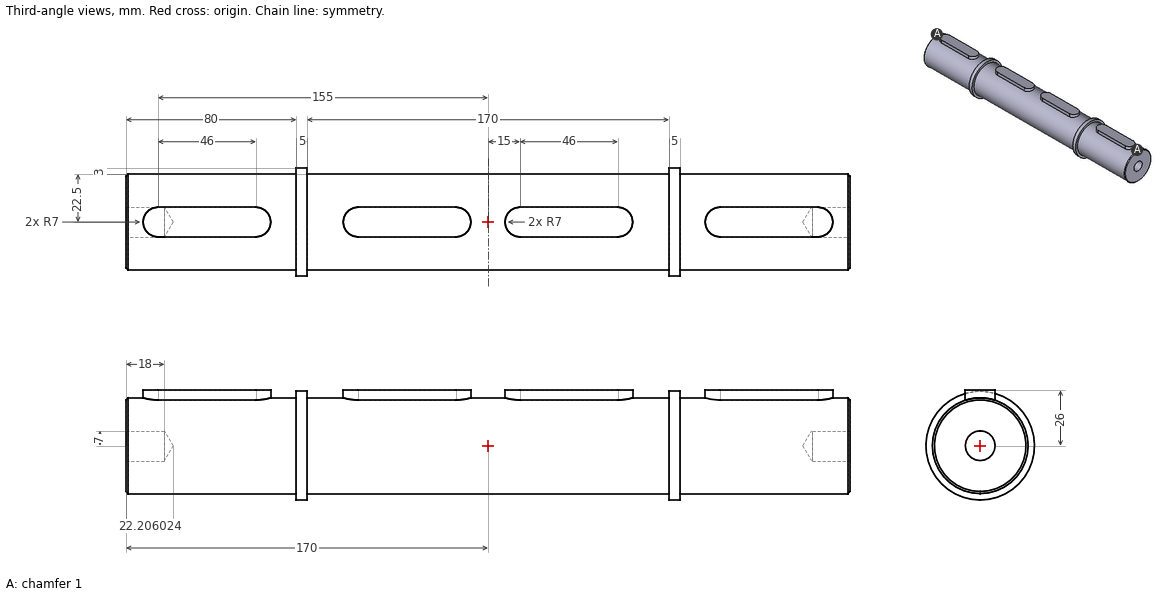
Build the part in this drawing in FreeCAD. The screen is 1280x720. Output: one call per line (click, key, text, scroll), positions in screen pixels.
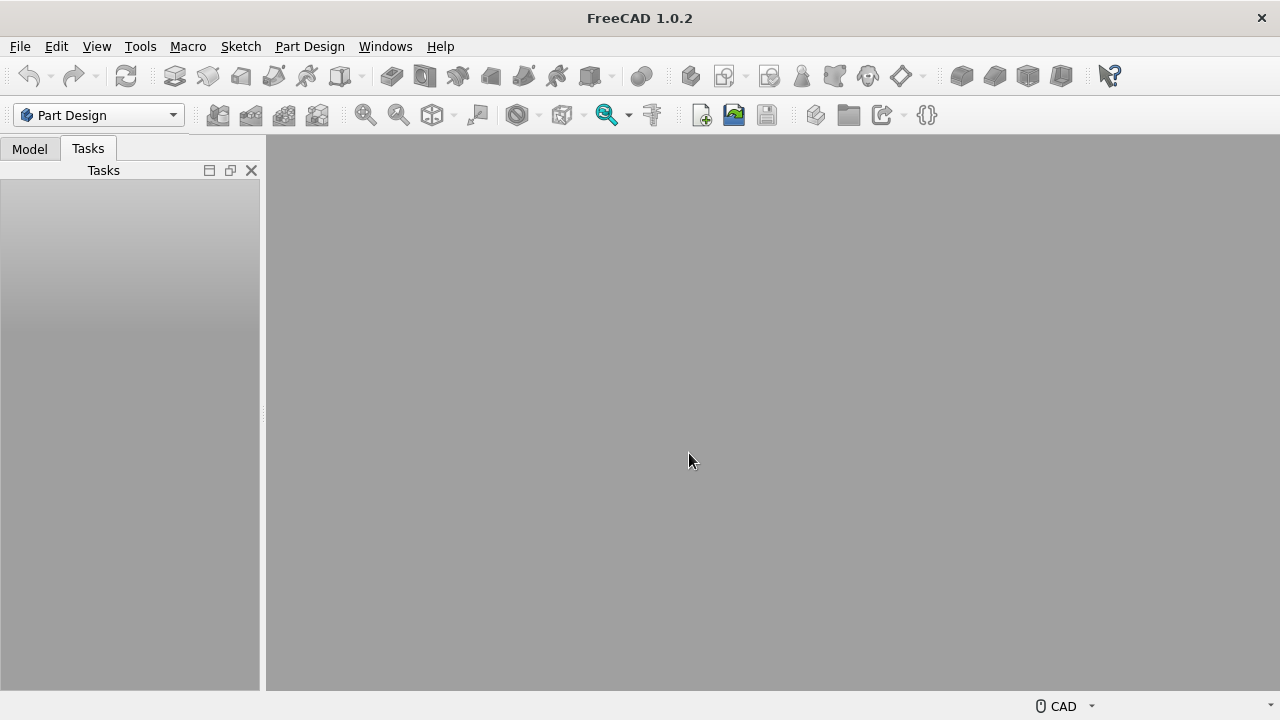
click(701, 116)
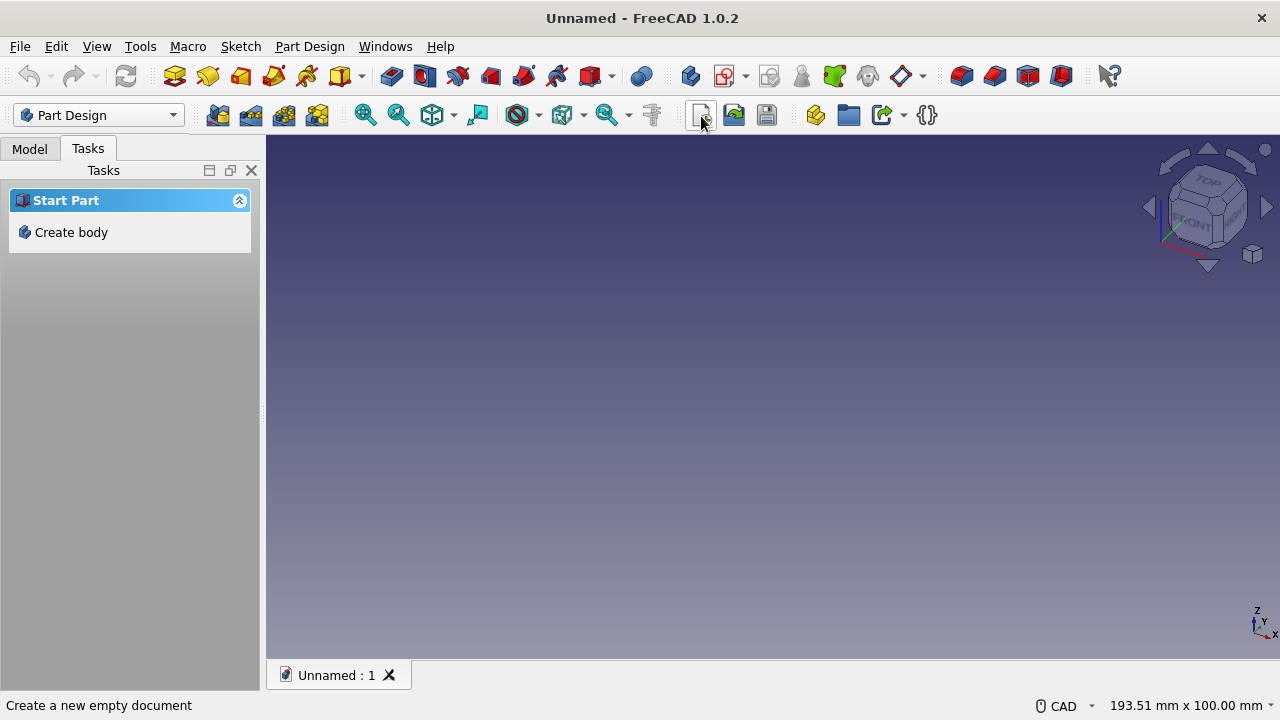
click(724, 76)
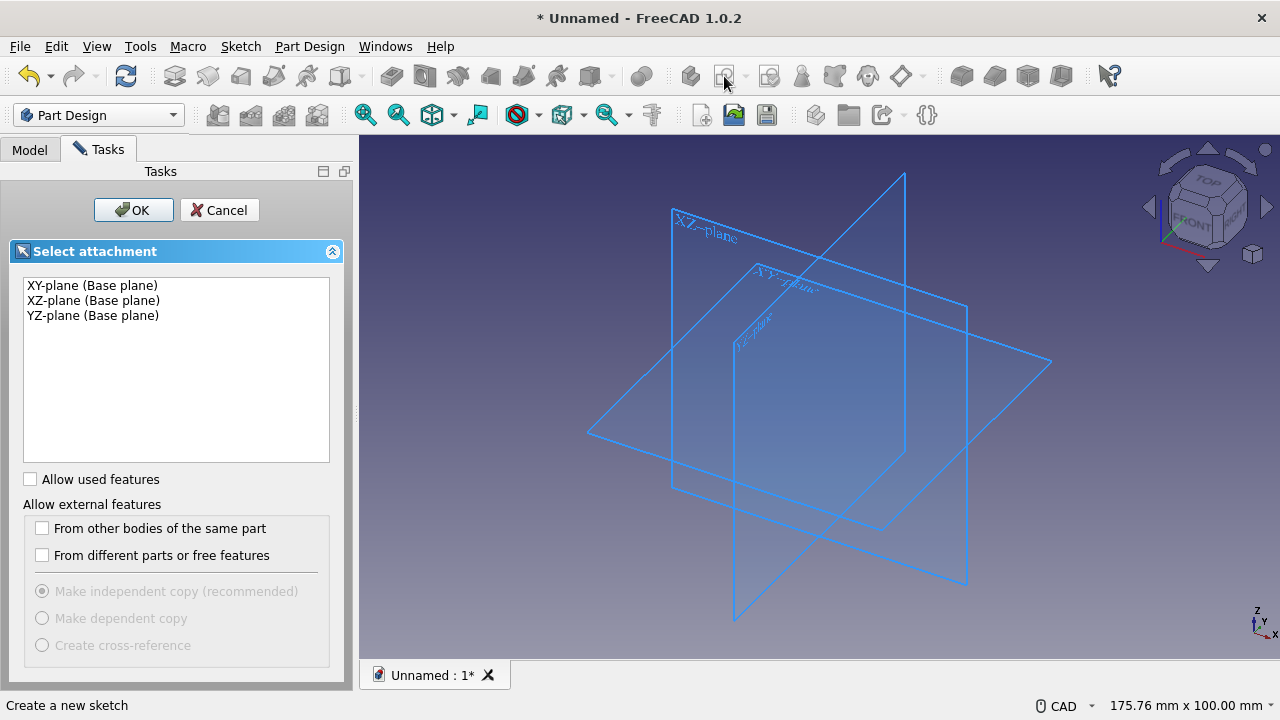
click(84, 286)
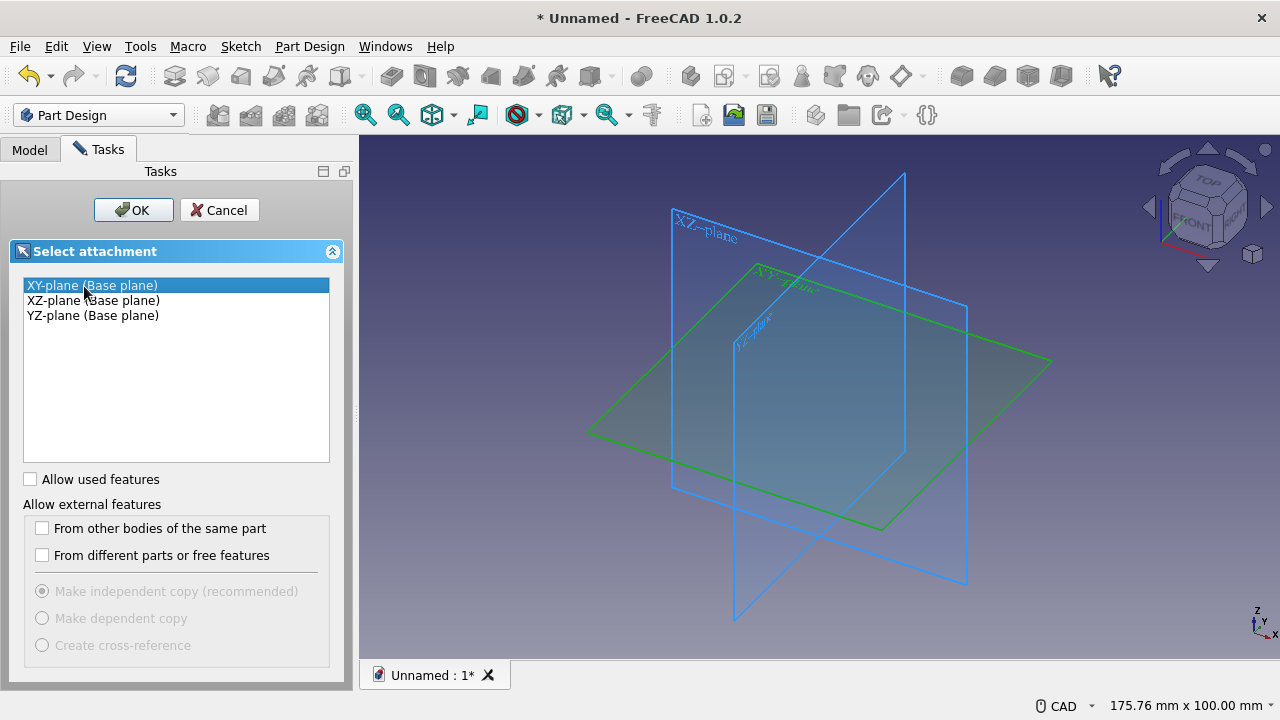
click(134, 210)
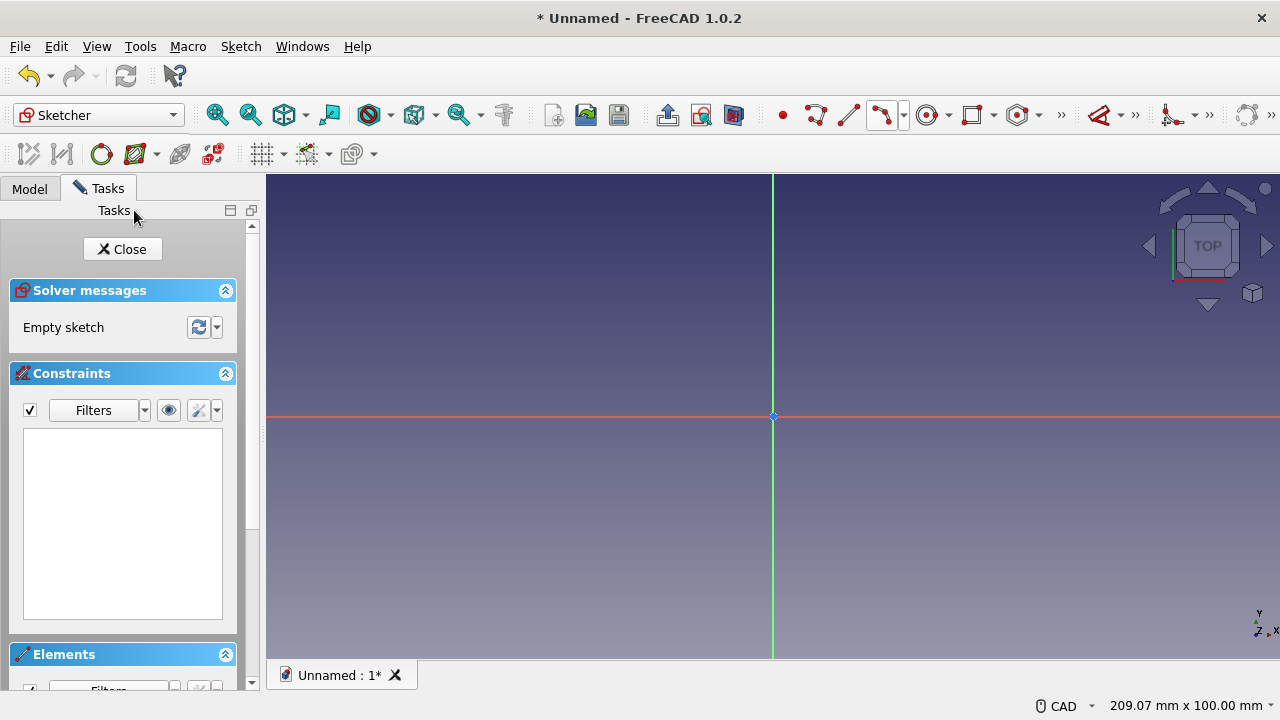
scroll(665, 452, down, 5)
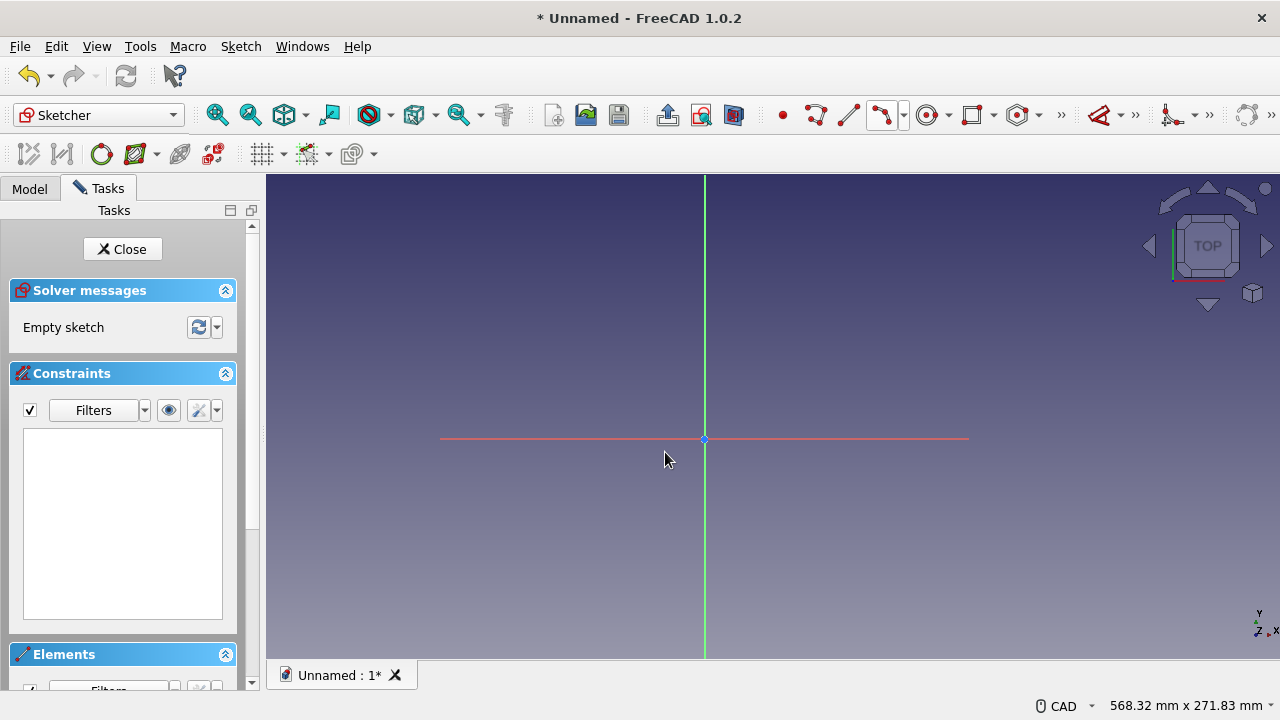
key(g)
key(m)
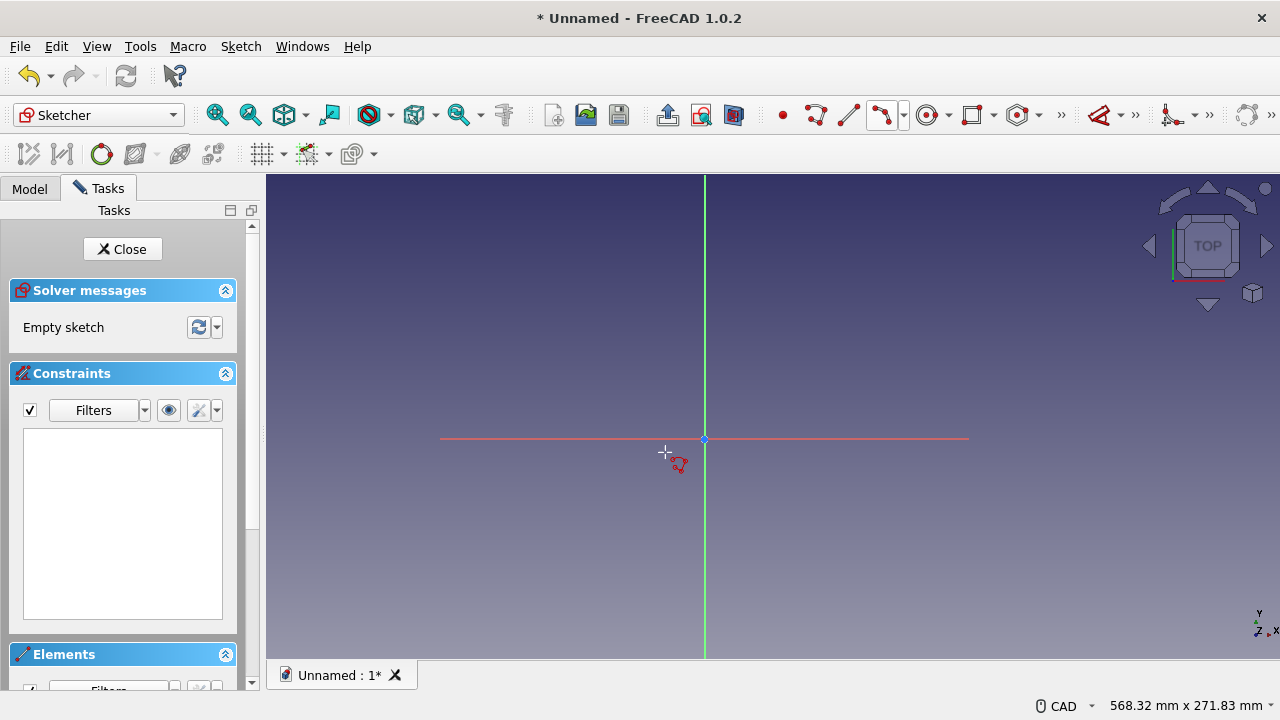
click(857, 399)
click(553, 399)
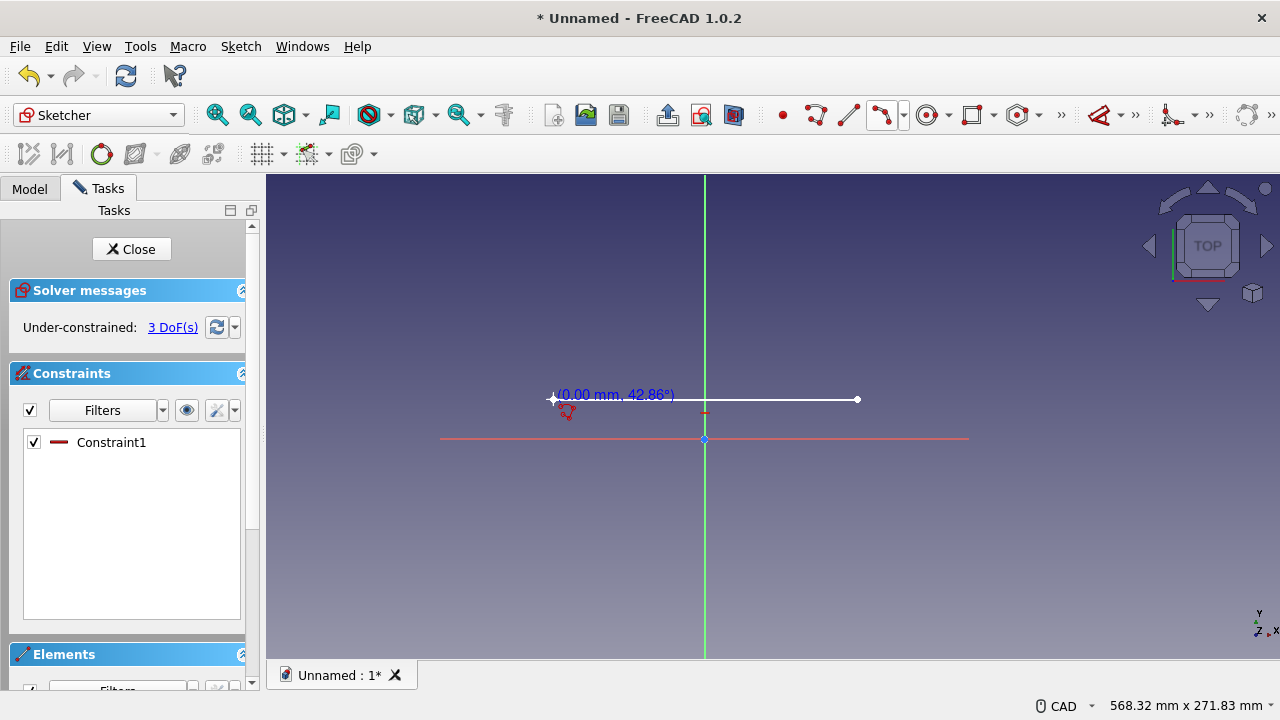
scroll(553, 394, up, 6)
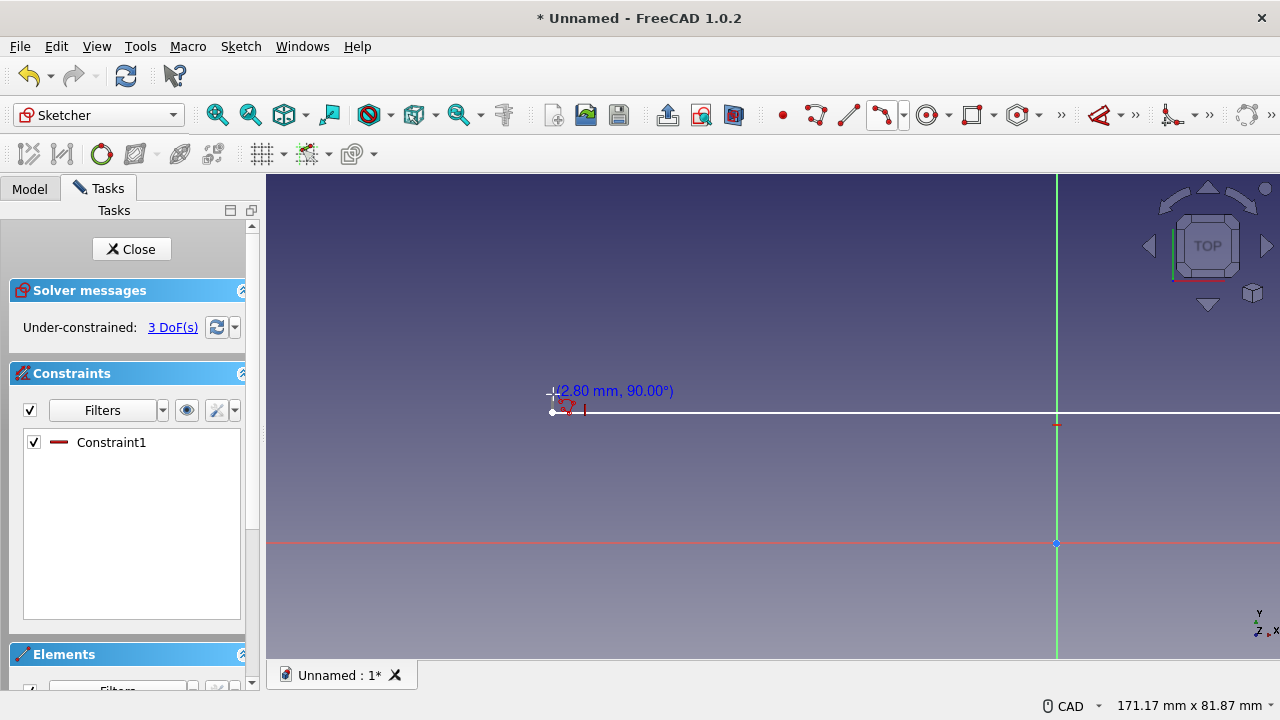
click(552, 392)
click(524, 392)
click(524, 410)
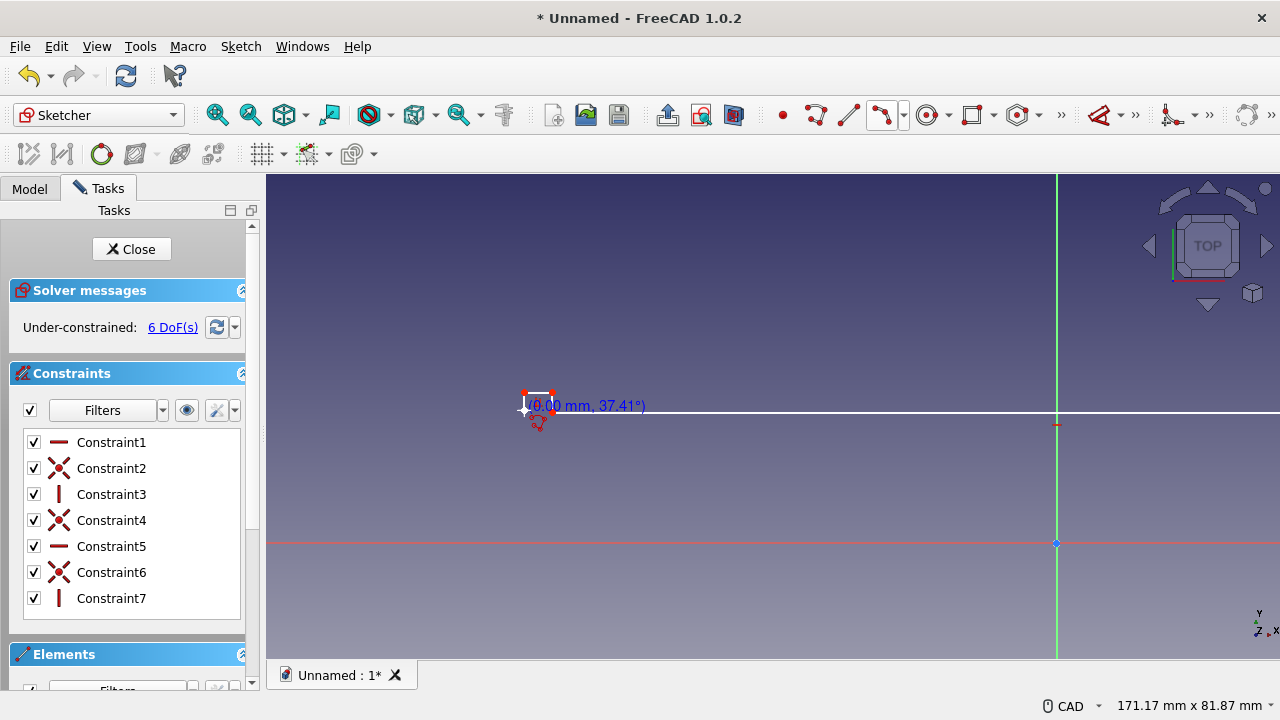
scroll(553, 394, down, 6)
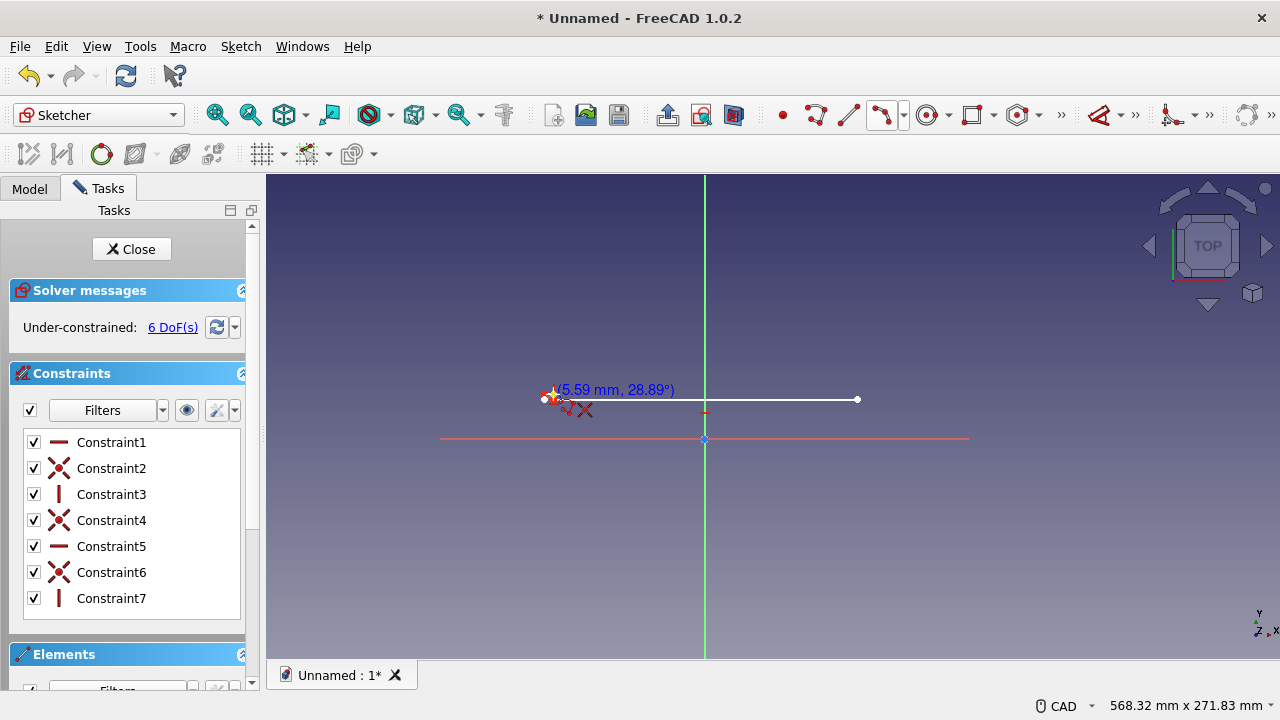
click(402, 399)
click(402, 439)
click(1008, 430)
click(1008, 399)